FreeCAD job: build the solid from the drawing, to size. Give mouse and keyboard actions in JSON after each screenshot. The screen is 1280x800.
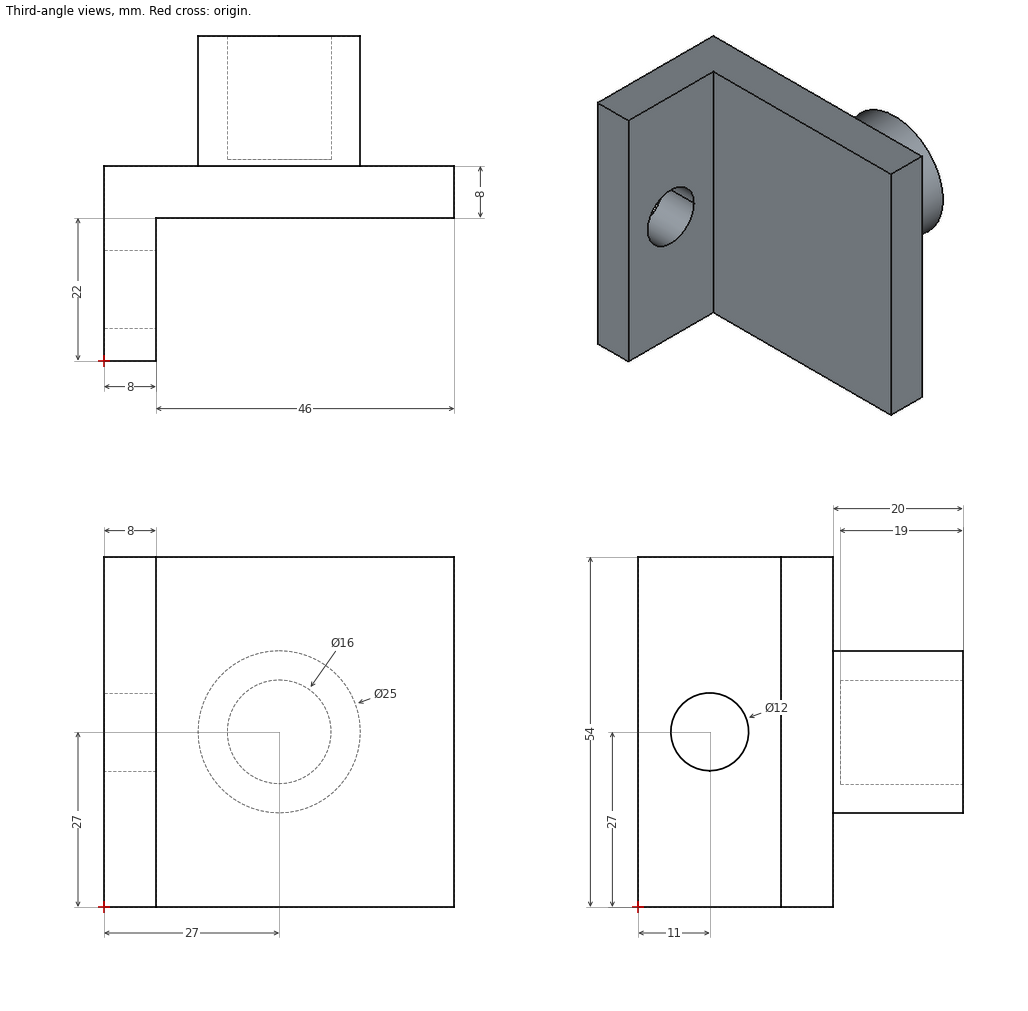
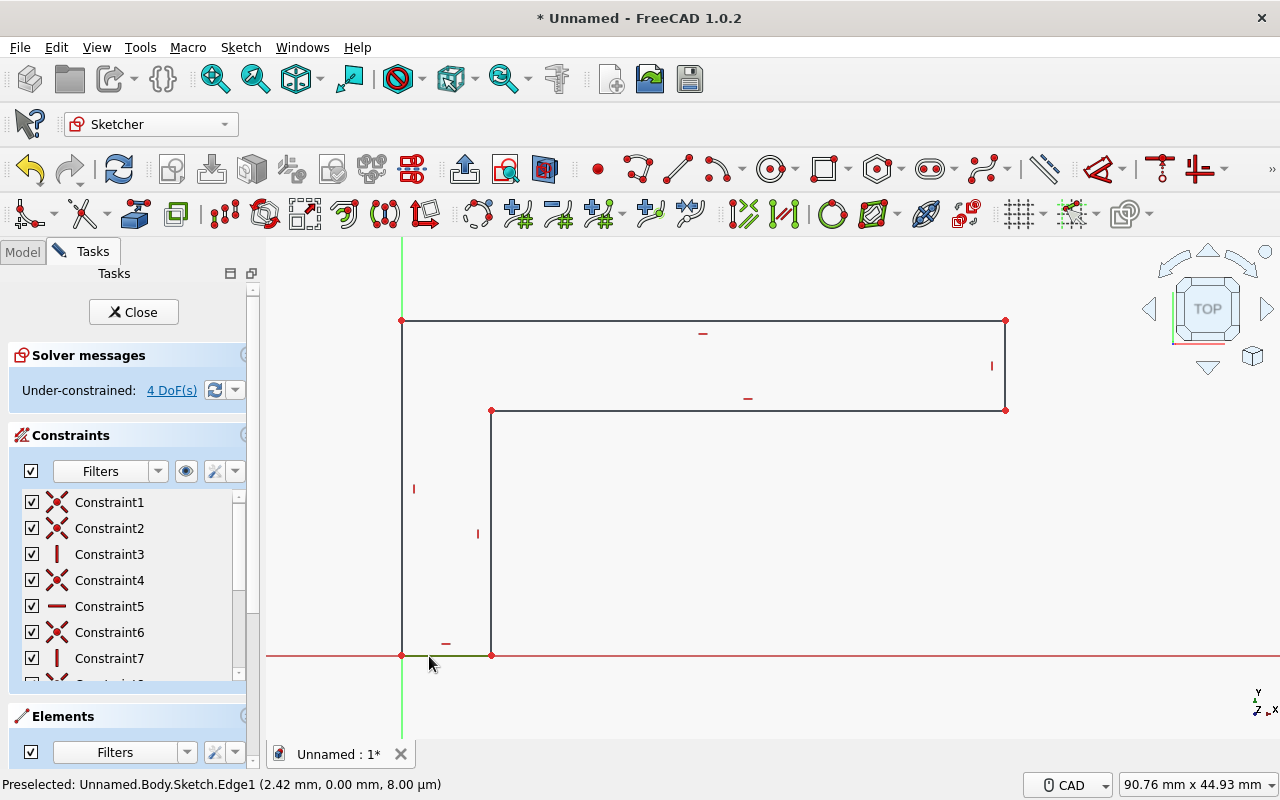
{"action": "key", "text": "l"}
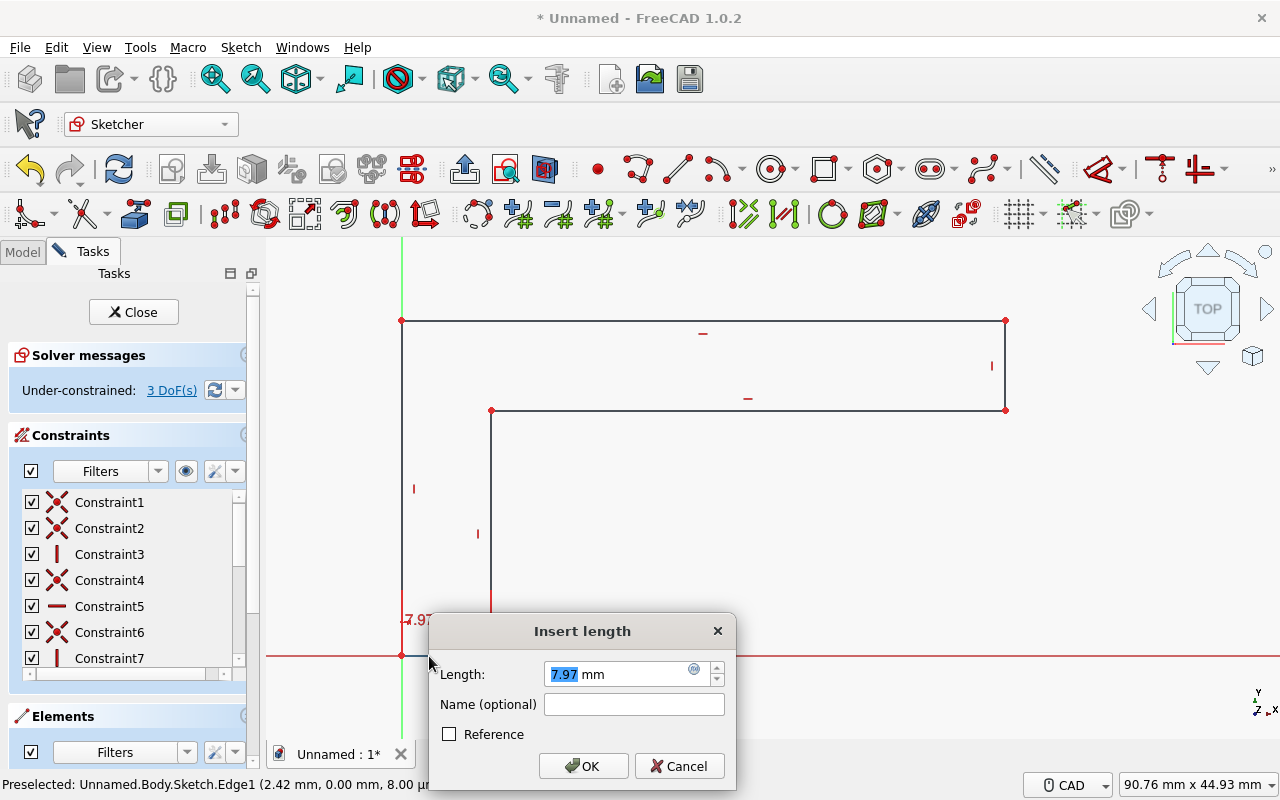
{"action": "type", "text": "8"}
{"action": "key", "text": "Return"}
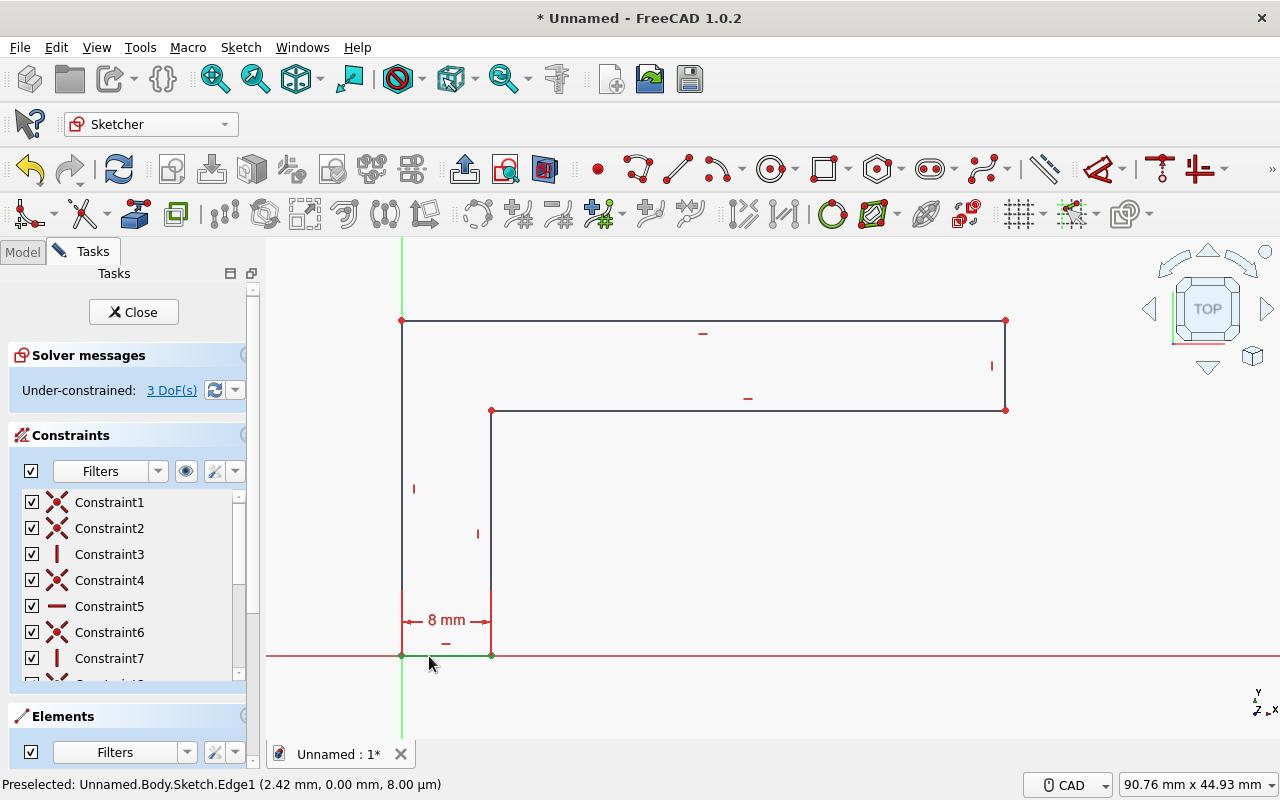
{"action": "left_click", "coordinate": [1005, 384]}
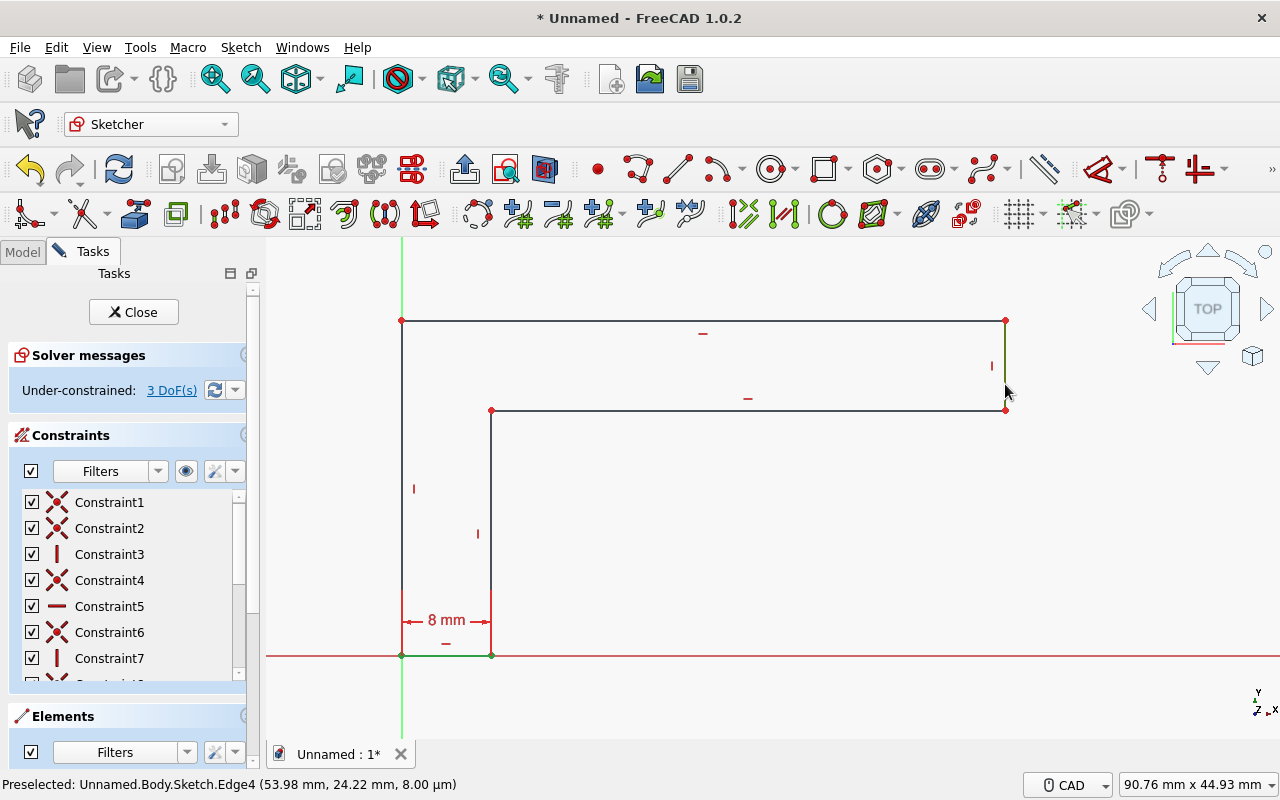
{"action": "left_click", "coordinate": [1124, 170]}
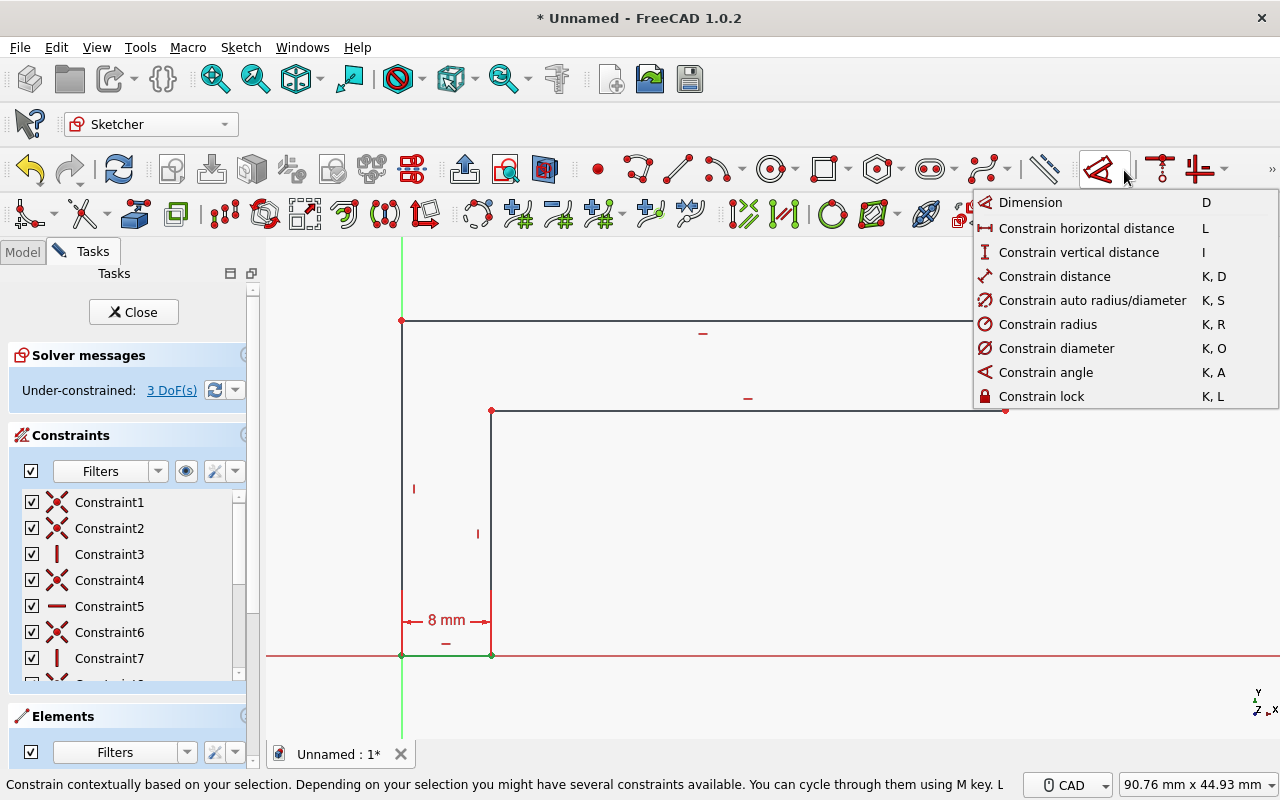
{"action": "left_click", "coordinate": [1126, 252]}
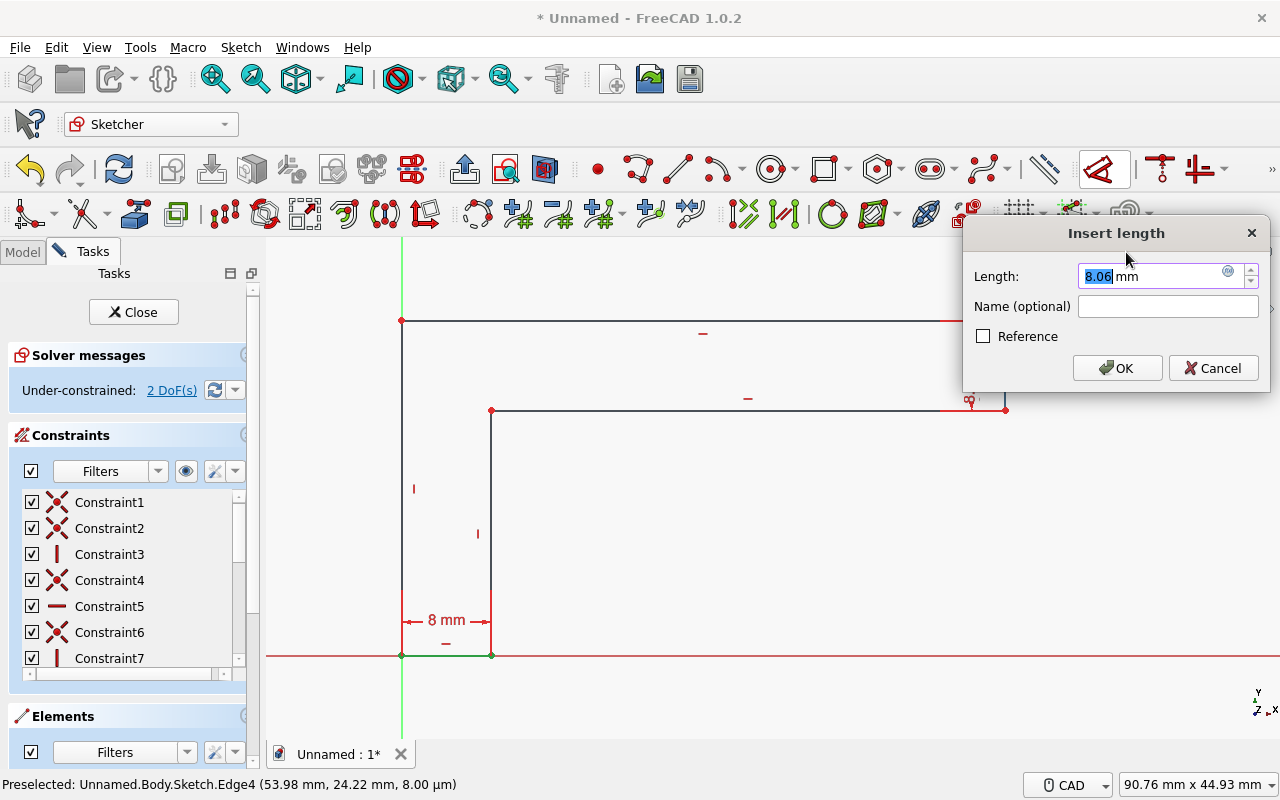
{"action": "type", "text": "8"}
{"action": "key", "text": "Return"}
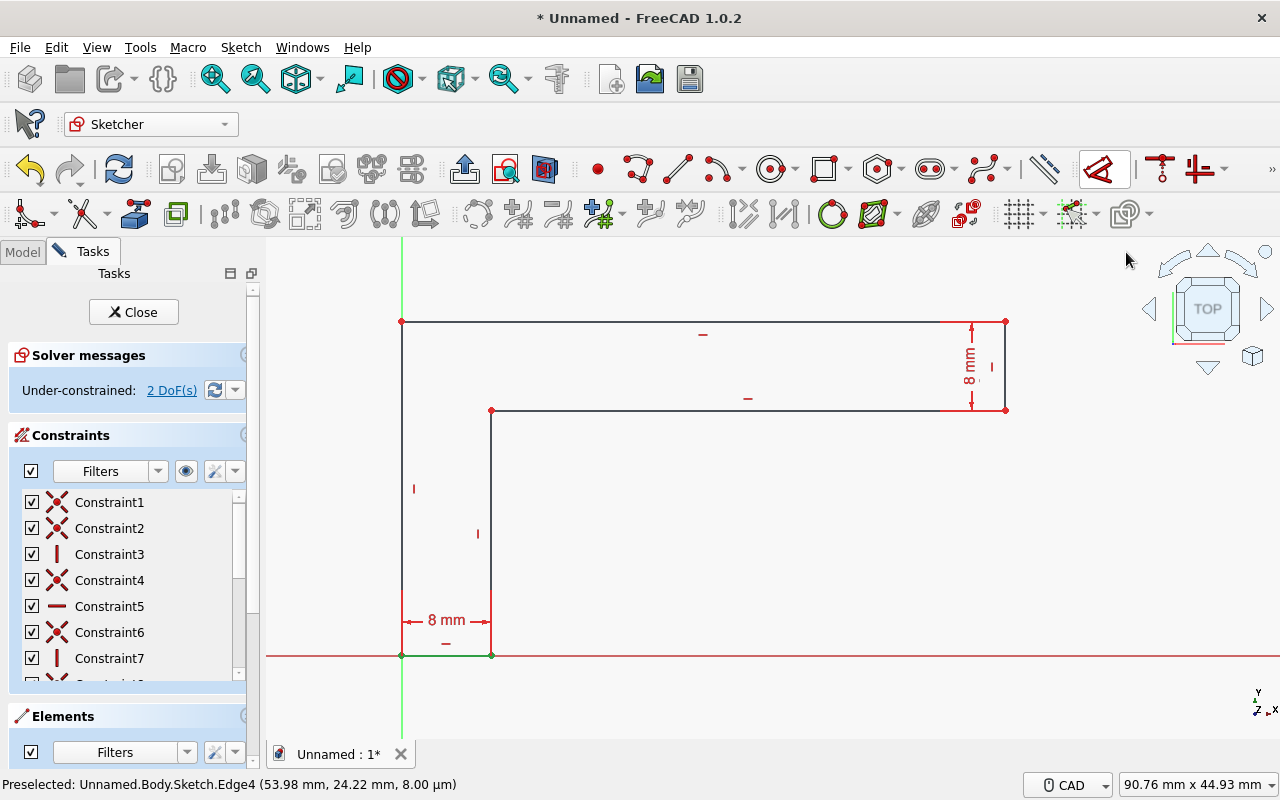
{"action": "left_click", "coordinate": [491, 582]}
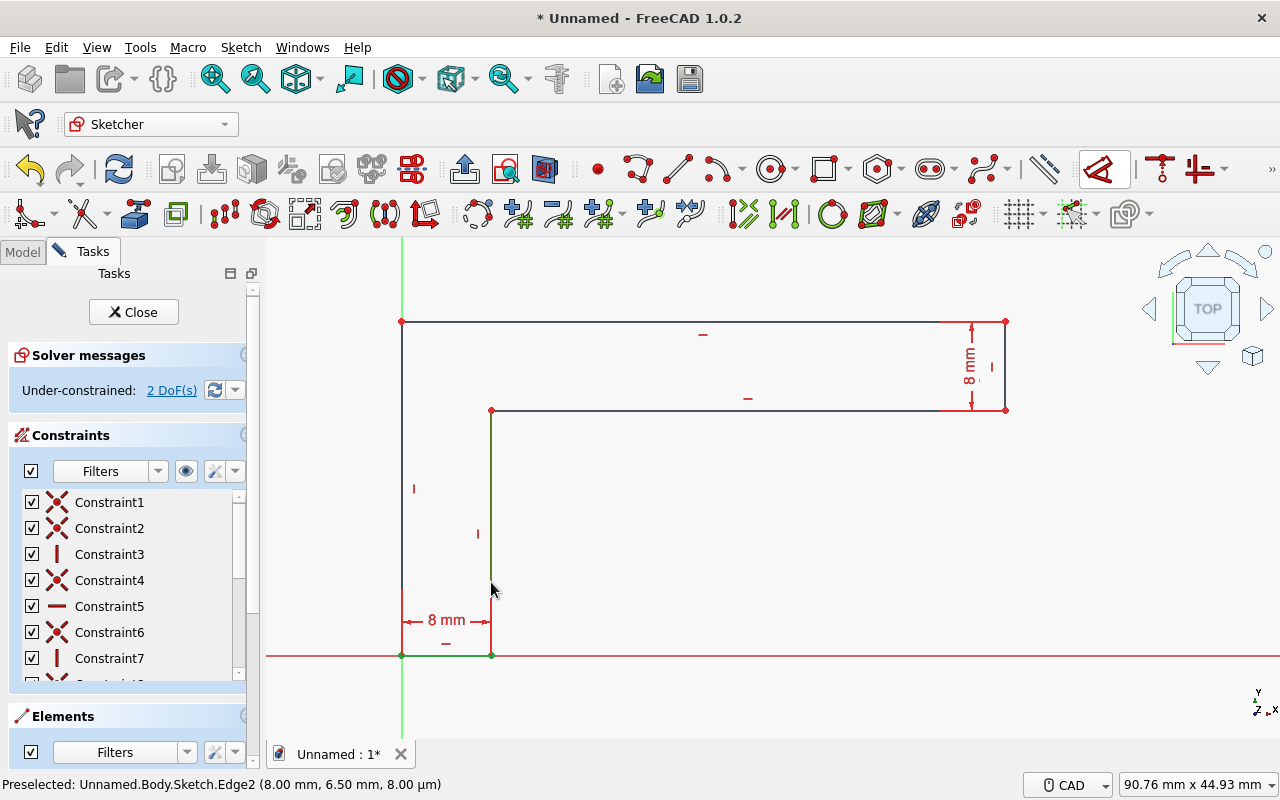
{"action": "key", "text": "i"}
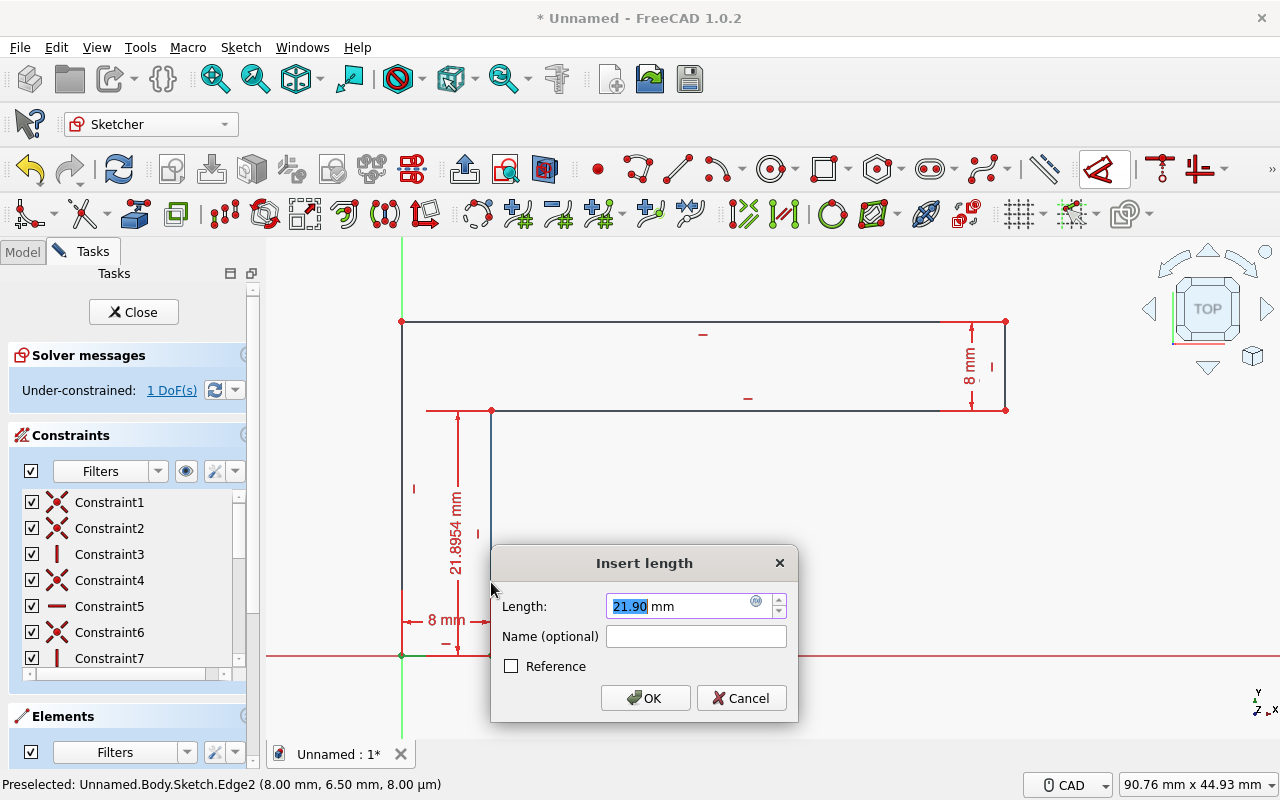
{"action": "type", "text": "22"}
{"action": "key", "text": "Return"}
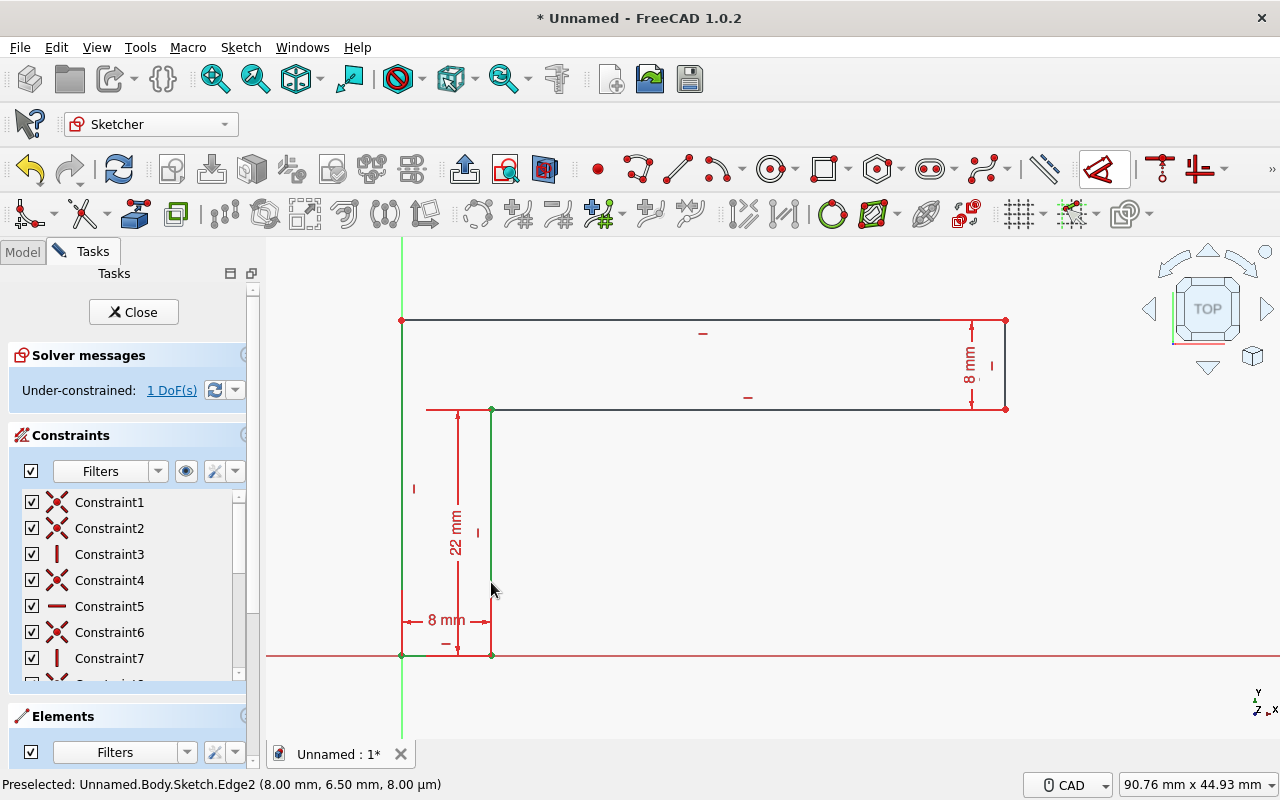
{"action": "left_click", "coordinate": [645, 410]}